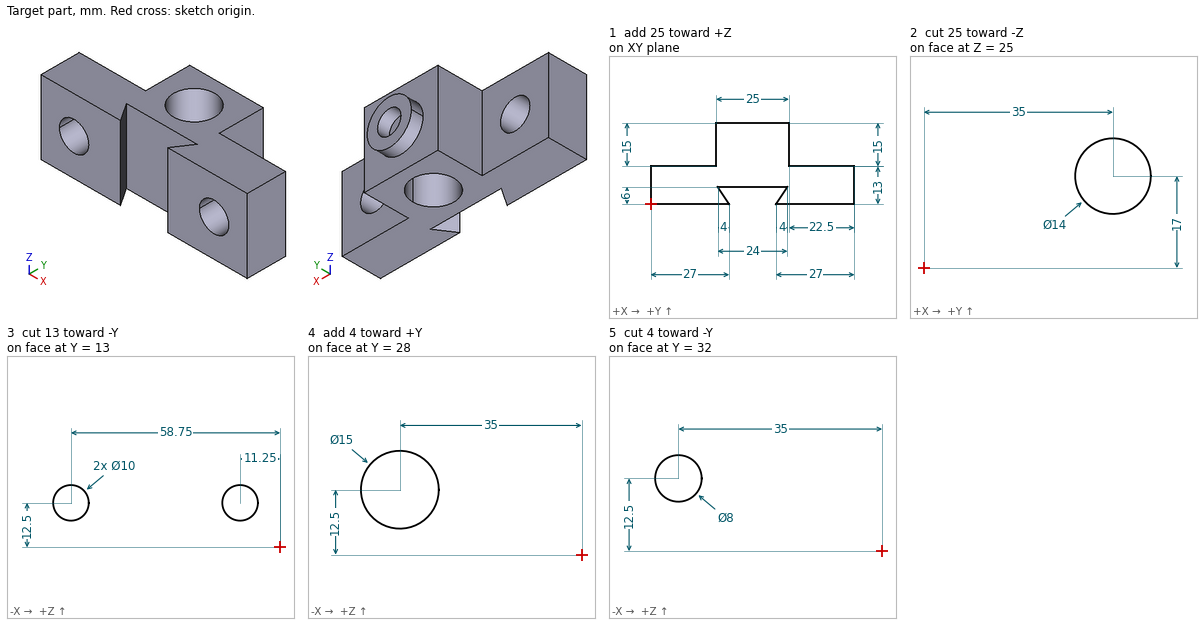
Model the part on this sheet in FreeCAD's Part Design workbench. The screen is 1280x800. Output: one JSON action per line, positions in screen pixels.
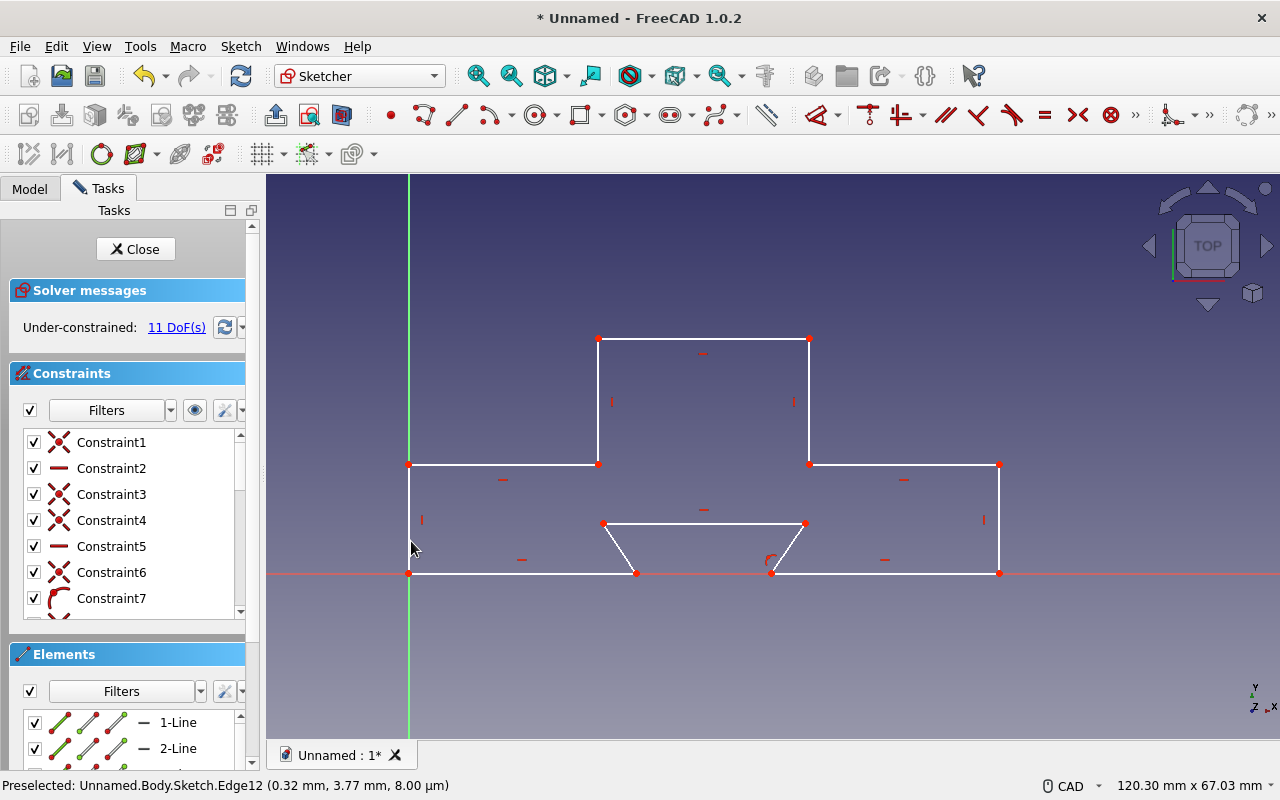
{"action": "left_click", "coordinate": [816, 116]}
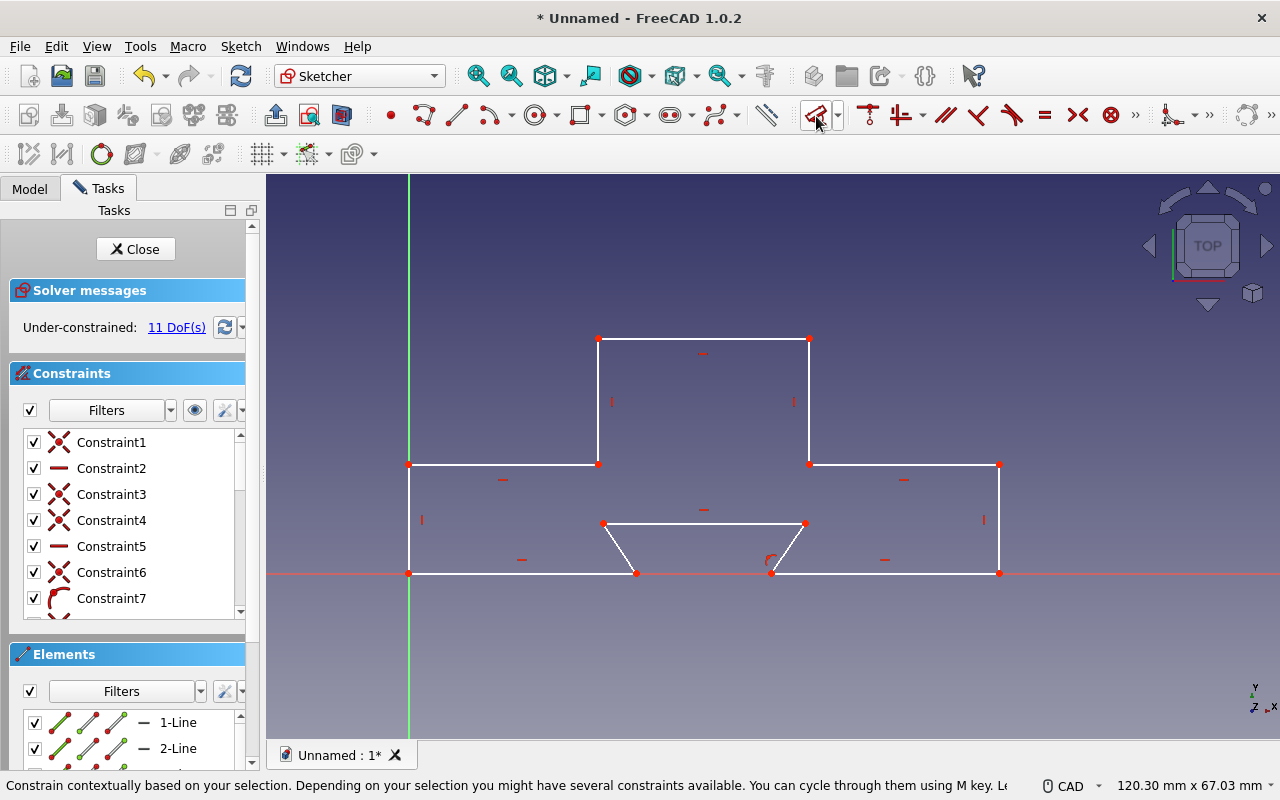
{"action": "left_click", "coordinate": [477, 574]}
{"action": "left_click", "coordinate": [522, 608]}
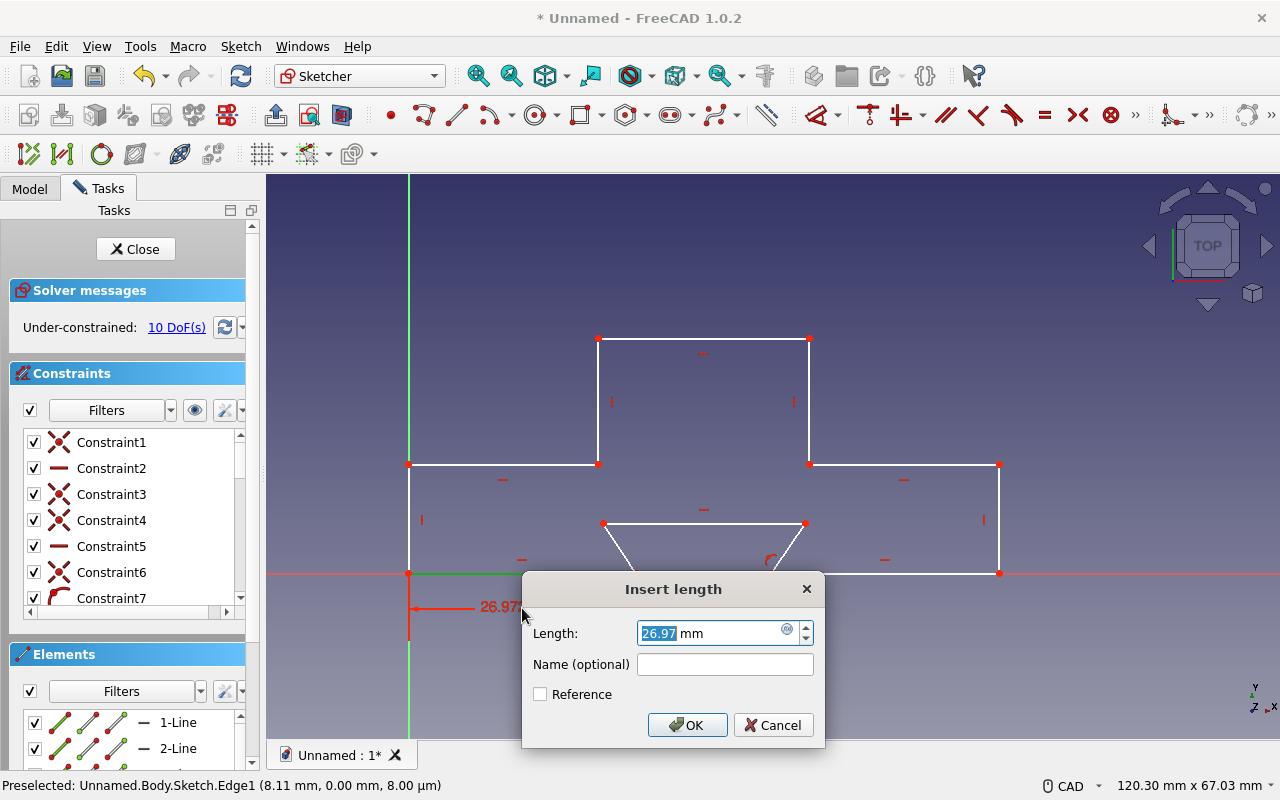
{"action": "type", "text": "27"}
{"action": "key", "text": "Return"}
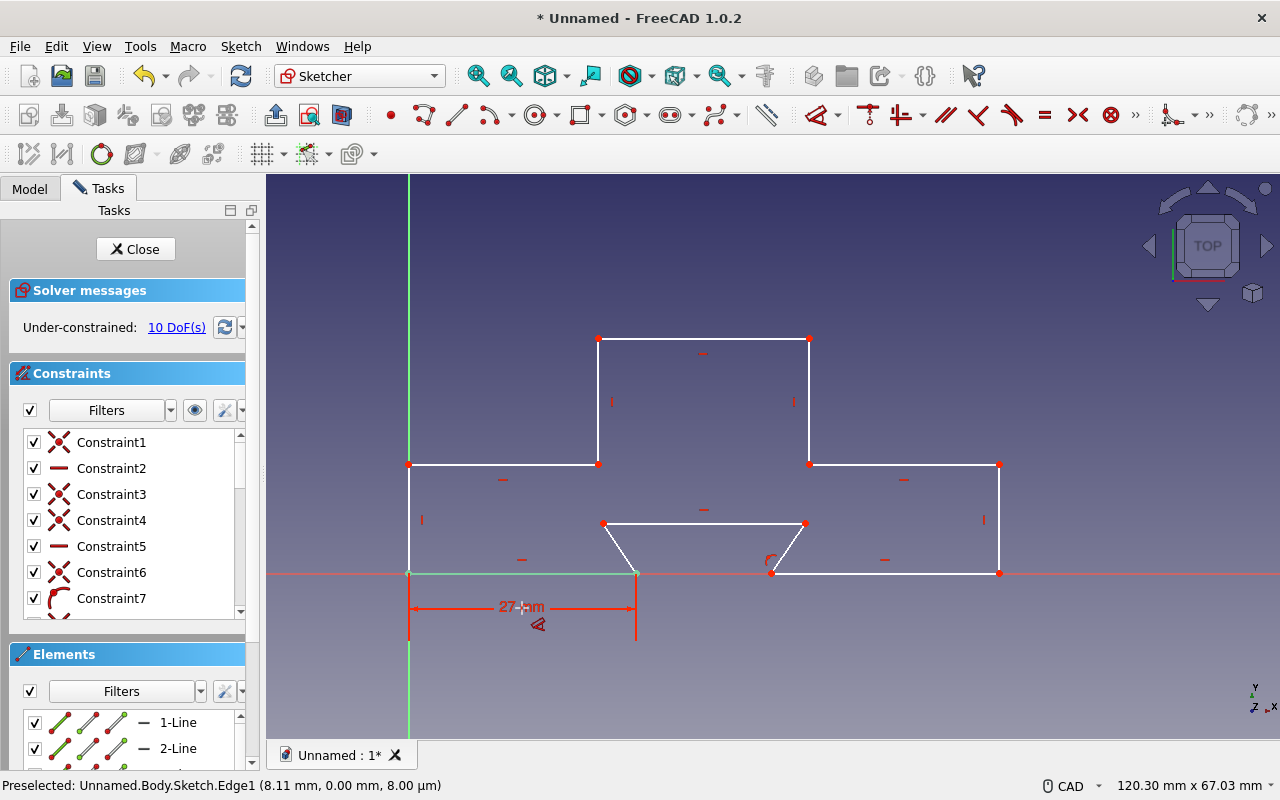
{"action": "left_click", "coordinate": [664, 524]}
{"action": "left_click", "coordinate": [704, 558]}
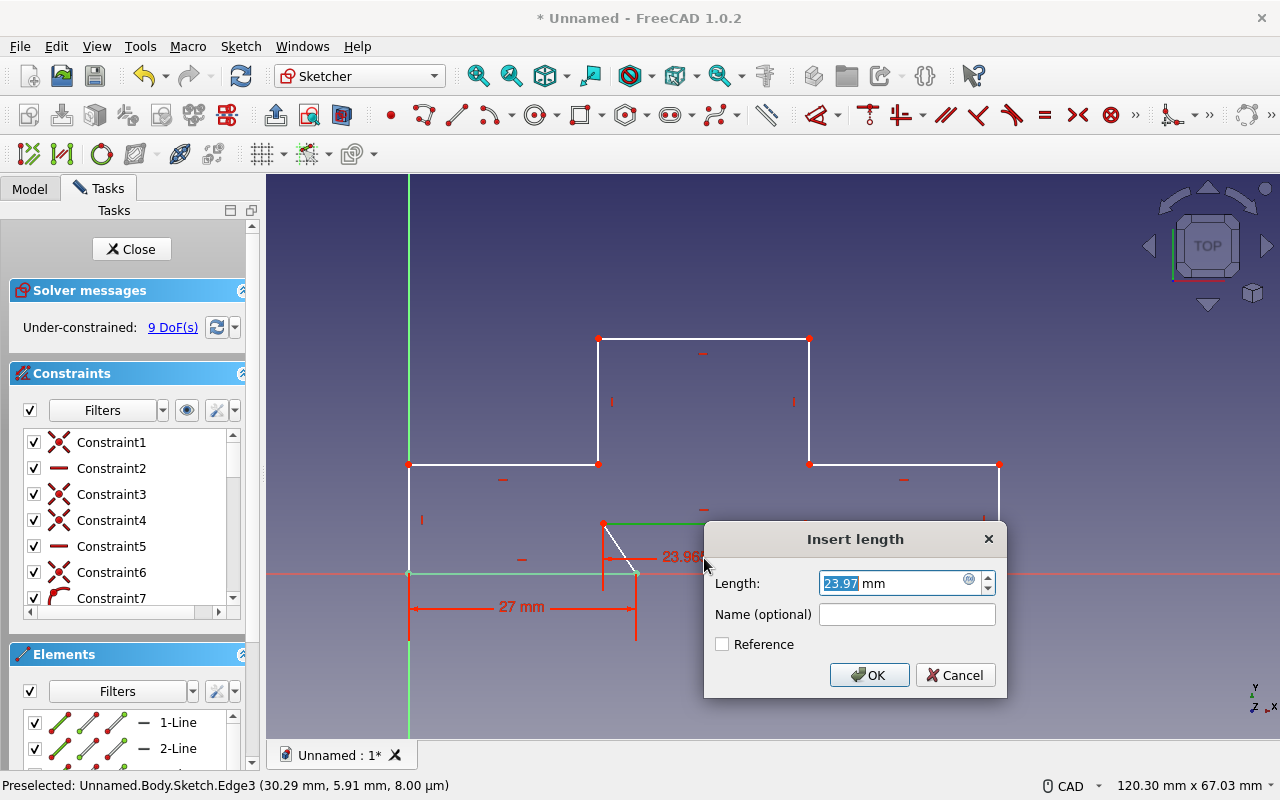
{"action": "type", "text": "24"}
{"action": "key", "text": "Return"}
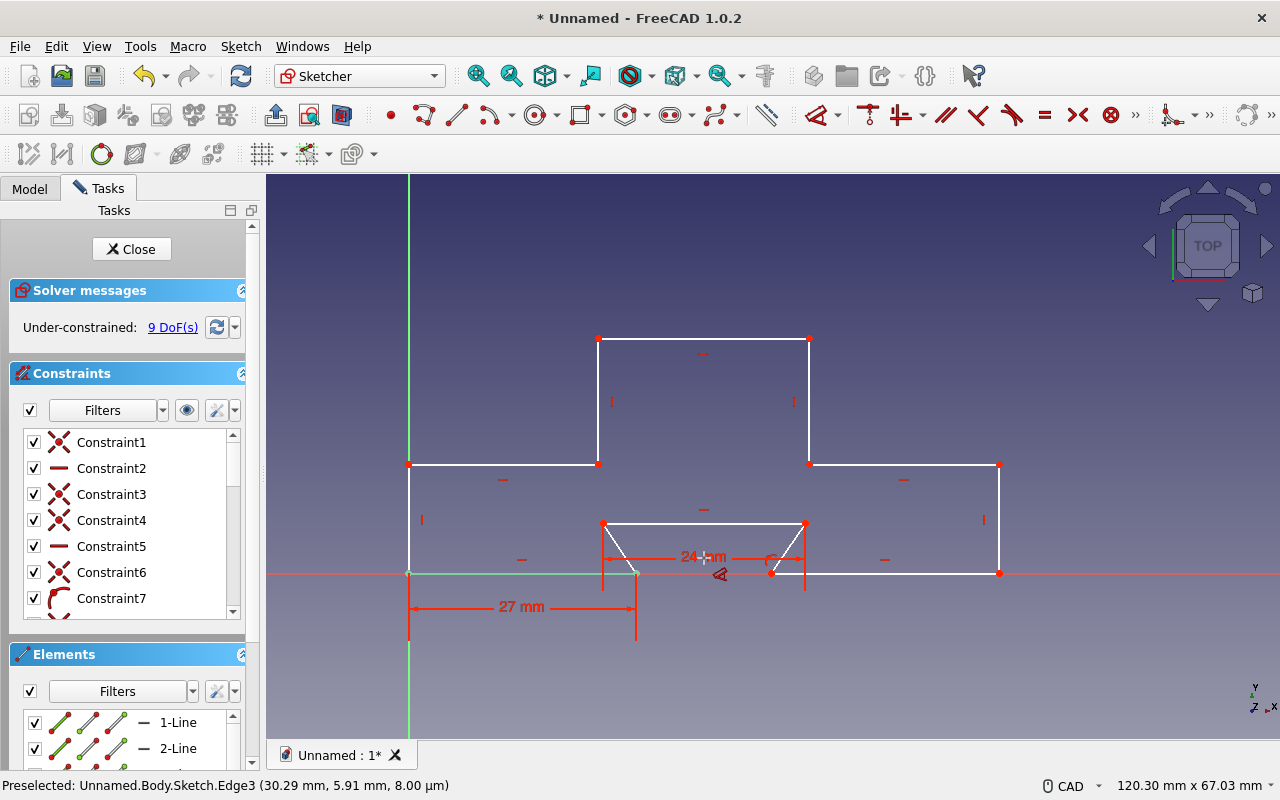
{"action": "left_click", "coordinate": [839, 574]}
{"action": "left_click", "coordinate": [885, 608]}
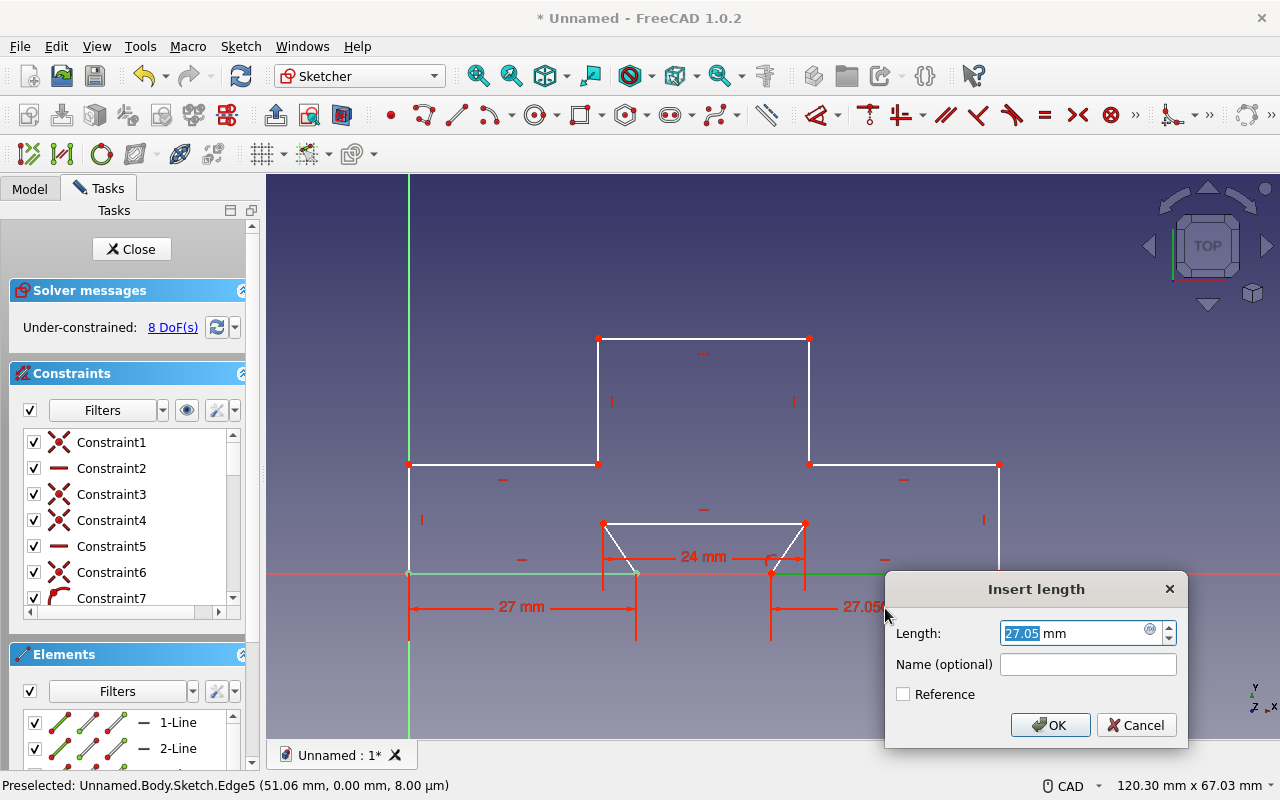
{"action": "type", "text": "27"}
{"action": "key", "text": "Return"}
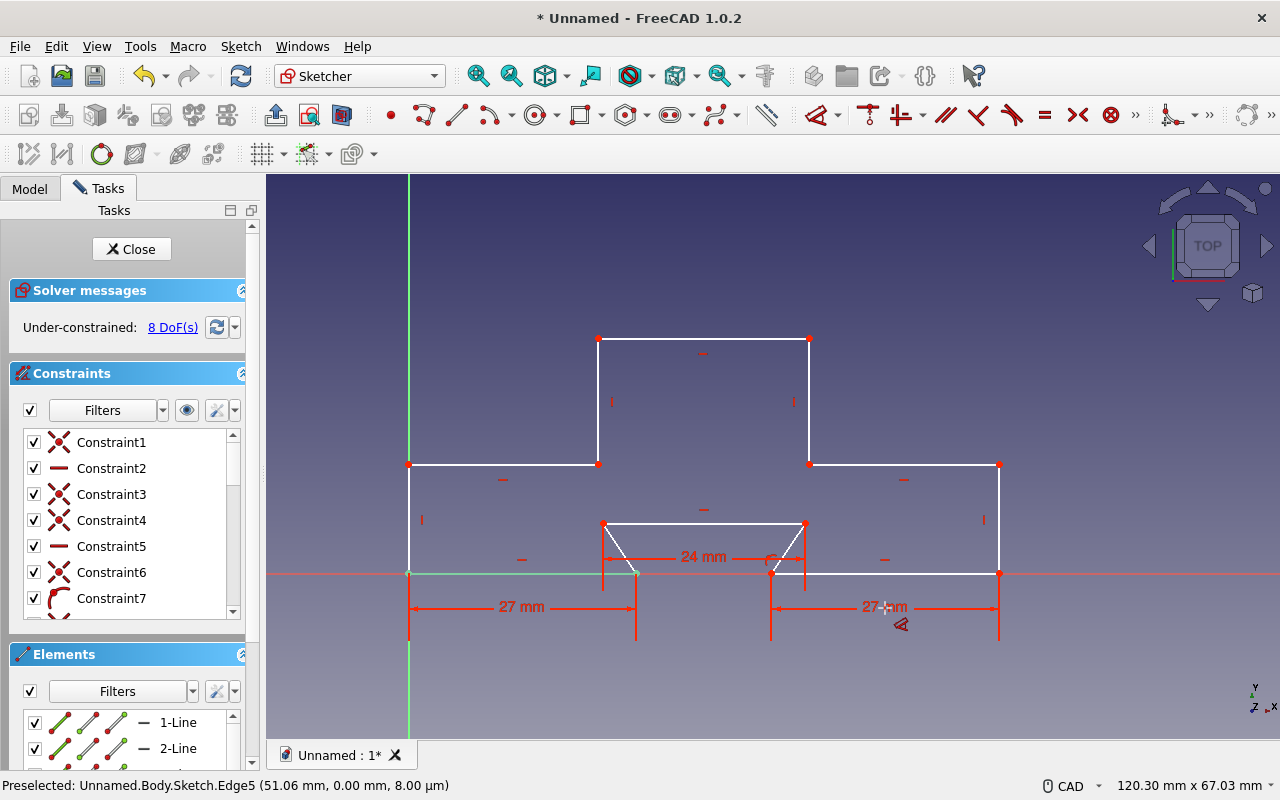
{"action": "left_click", "coordinate": [999, 541]}
{"action": "left_click", "coordinate": [1033, 519]}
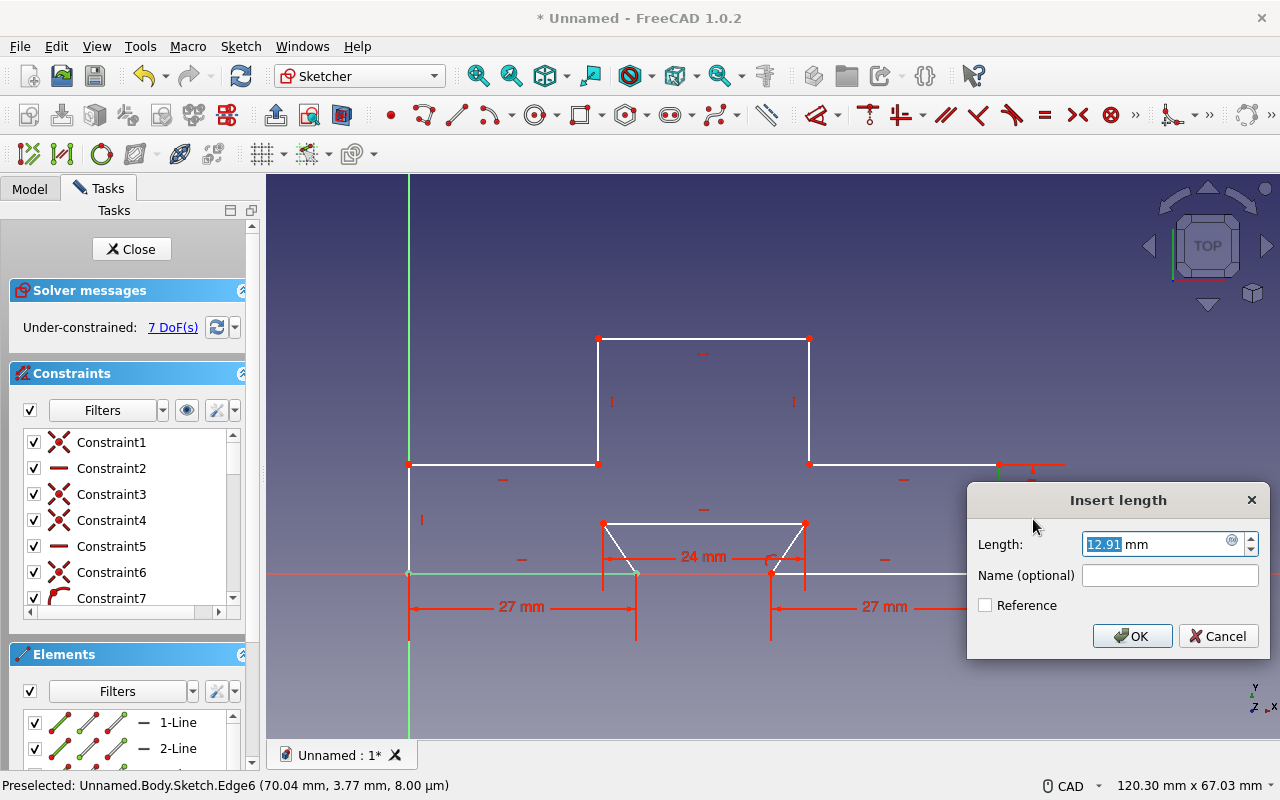
{"action": "type", "text": "13"}
{"action": "key", "text": "Return"}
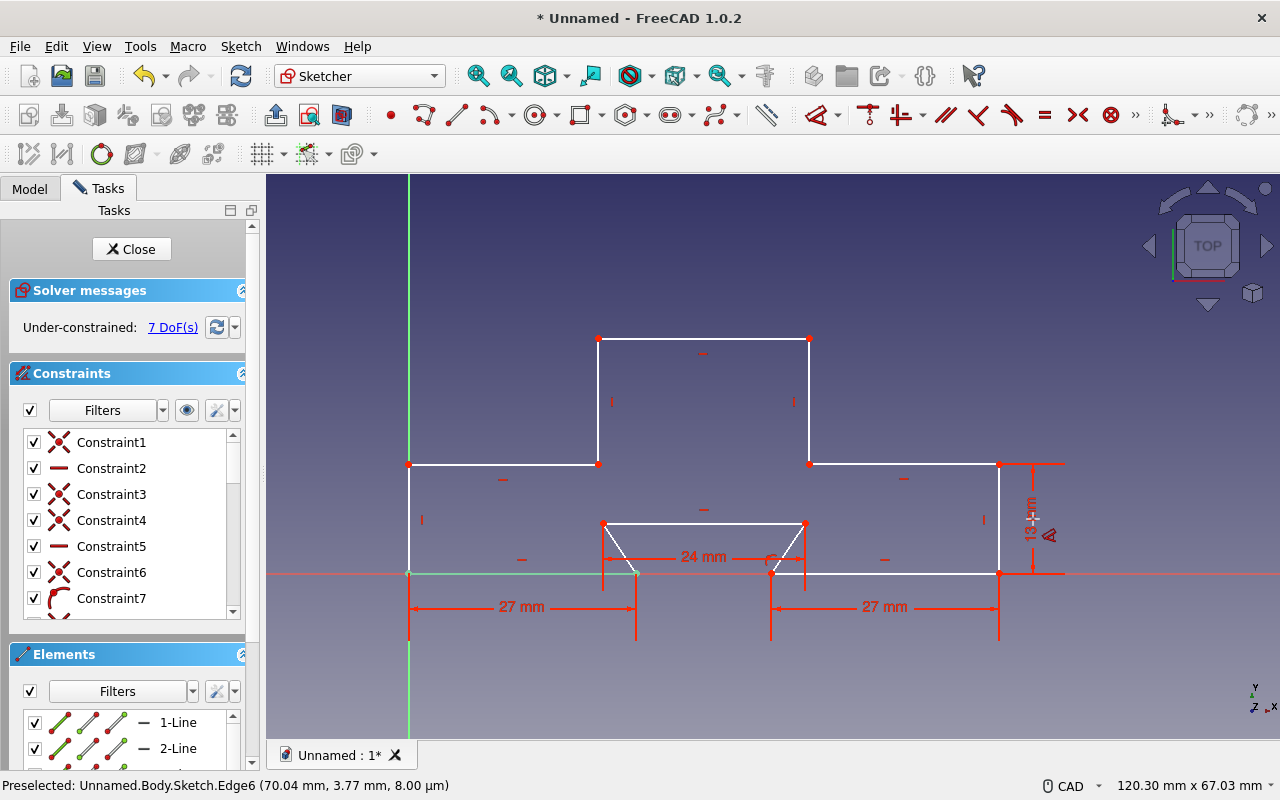
{"action": "left_click", "coordinate": [809, 427]}
{"action": "left_click", "coordinate": [843, 402]}